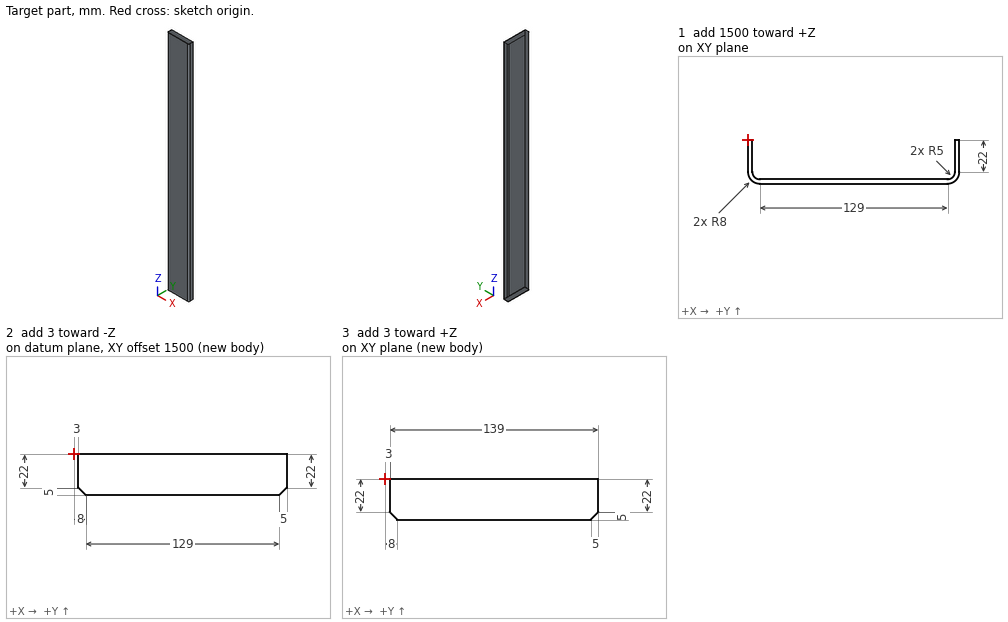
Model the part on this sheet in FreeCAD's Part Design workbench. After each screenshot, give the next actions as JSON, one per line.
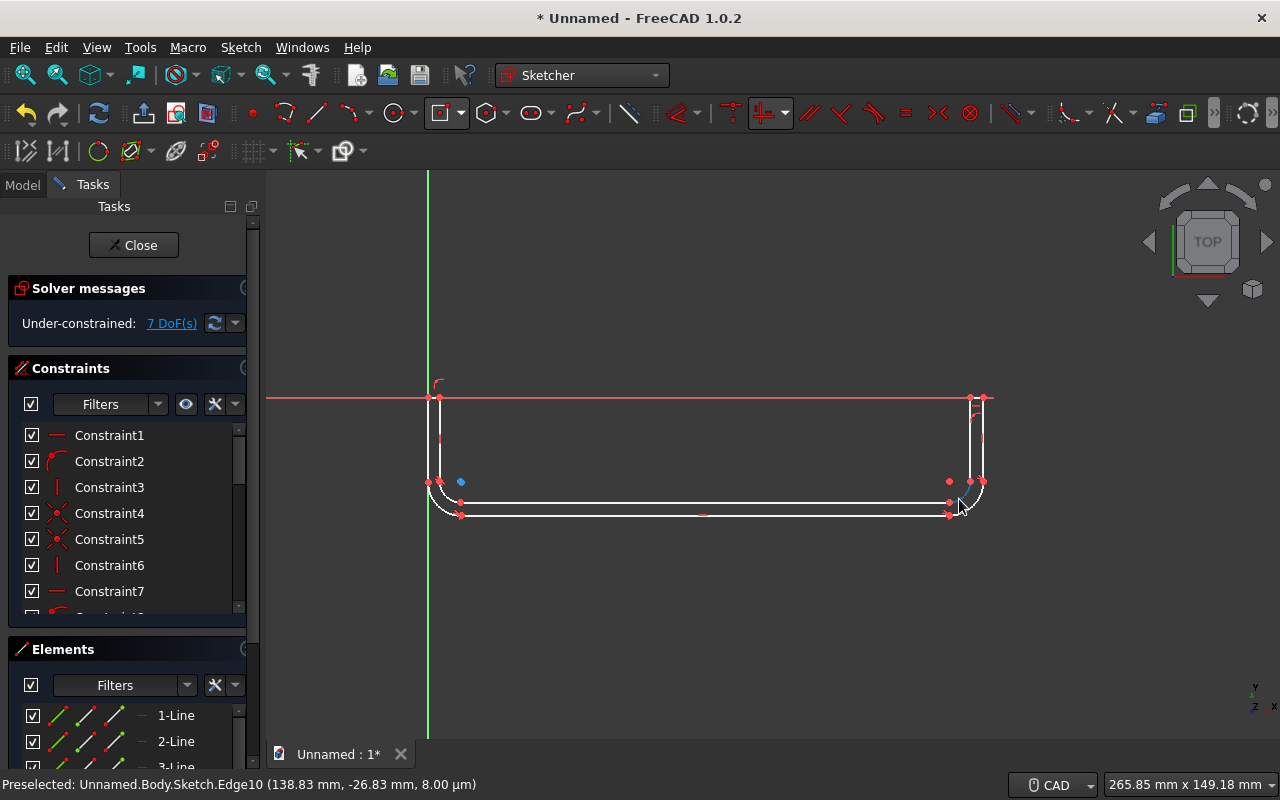
{"action": "scroll", "coordinate": [442, 491], "scroll_direction": "up", "scroll_amount": 2}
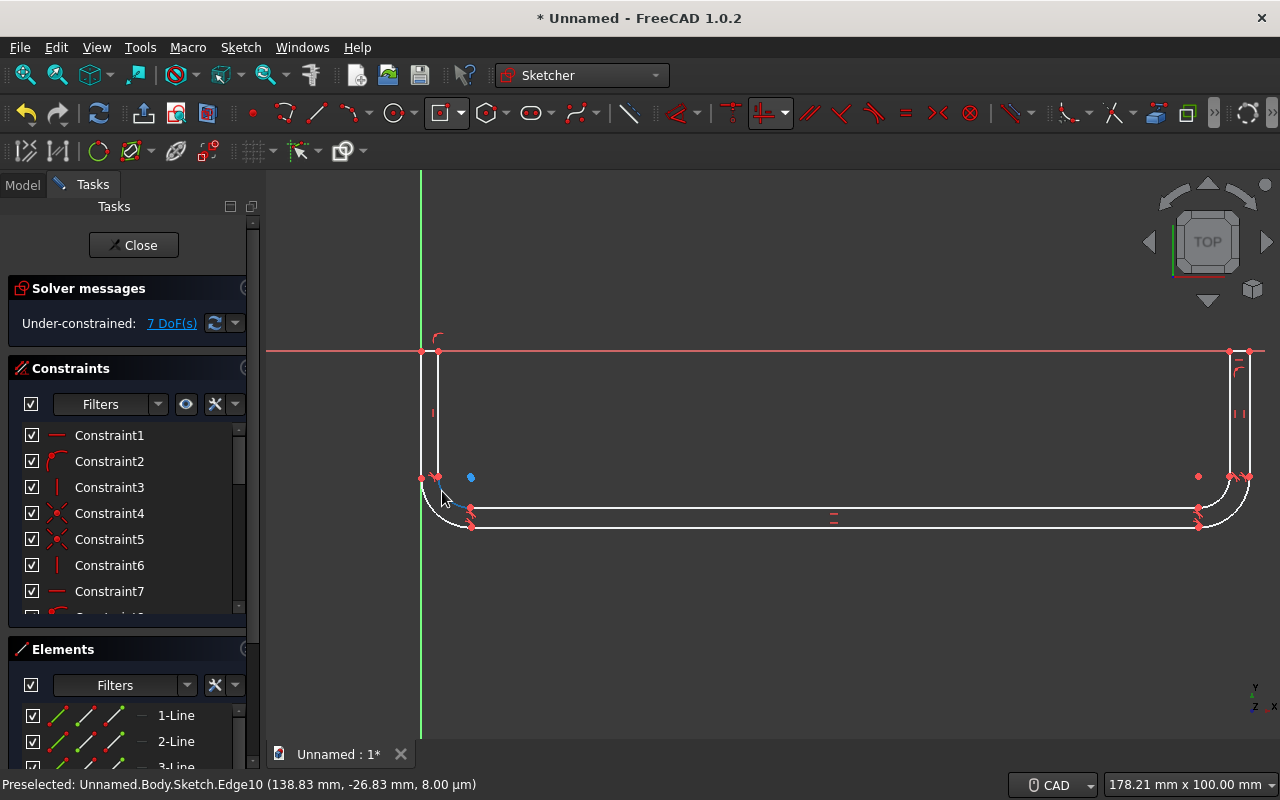
{"action": "left_click", "coordinate": [442, 490]}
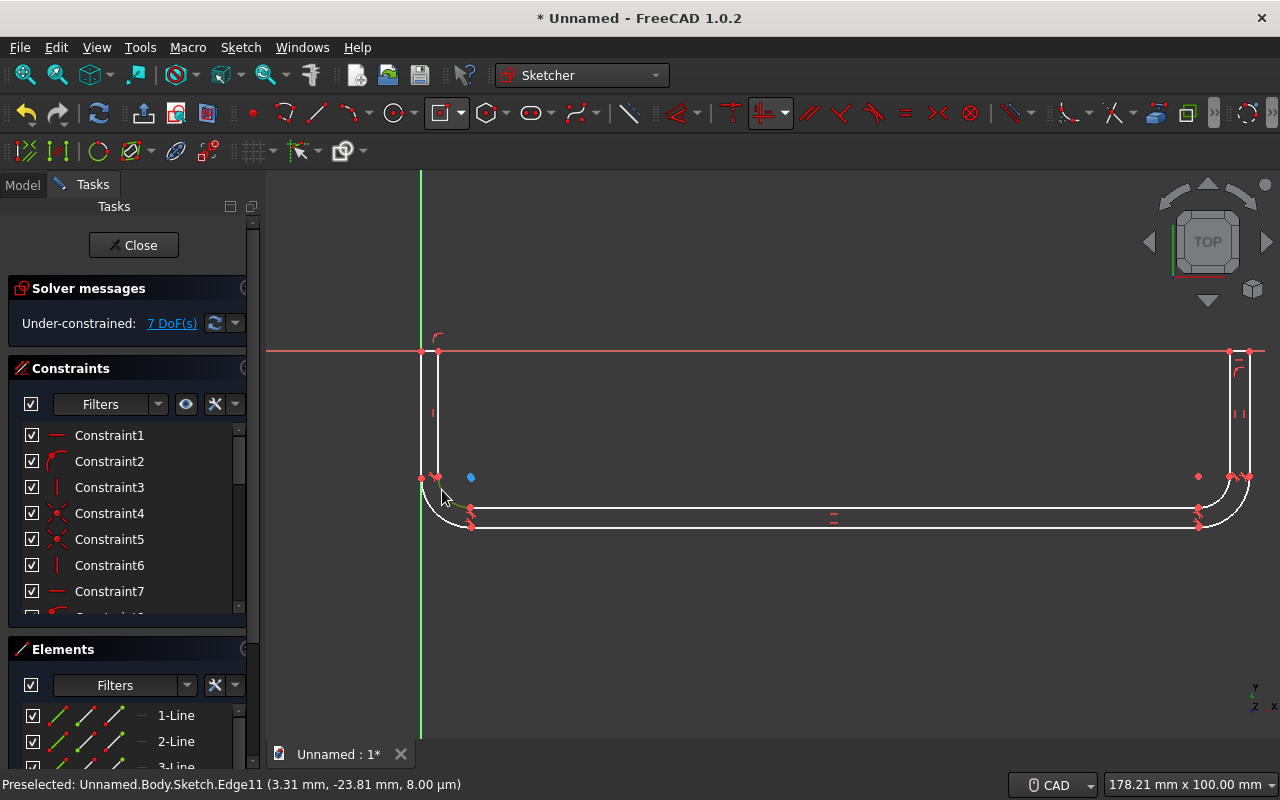
{"action": "left_click", "coordinate": [448, 522]}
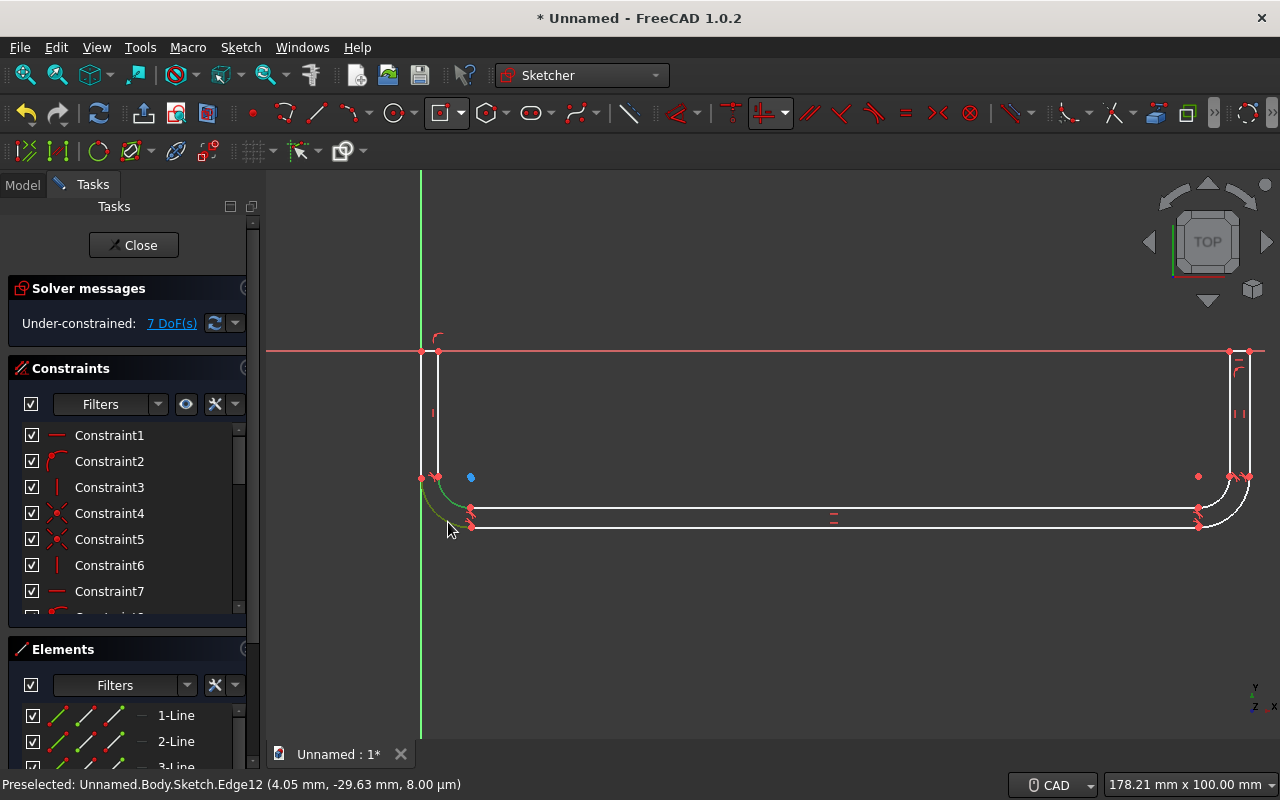
{"action": "left_click", "coordinate": [732, 114]}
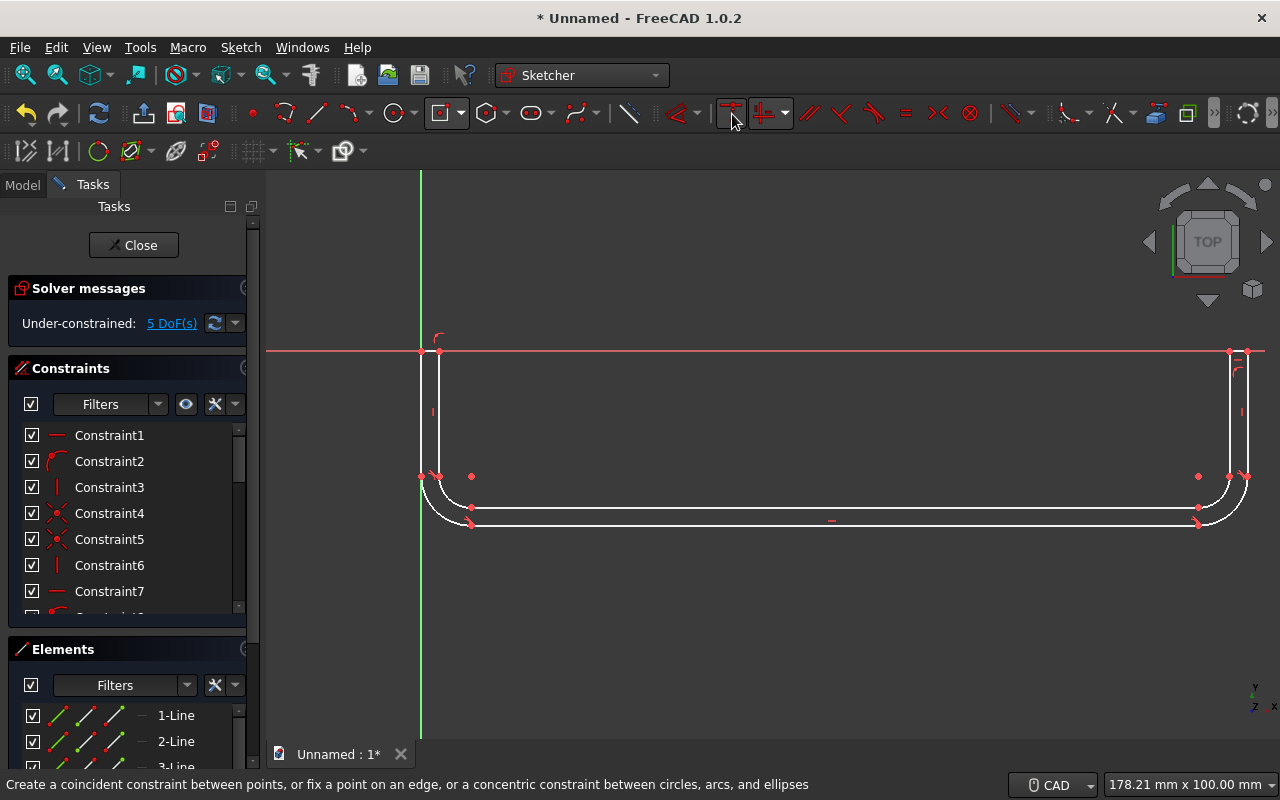
{"action": "scroll", "coordinate": [441, 491], "scroll_direction": "down", "scroll_amount": 2}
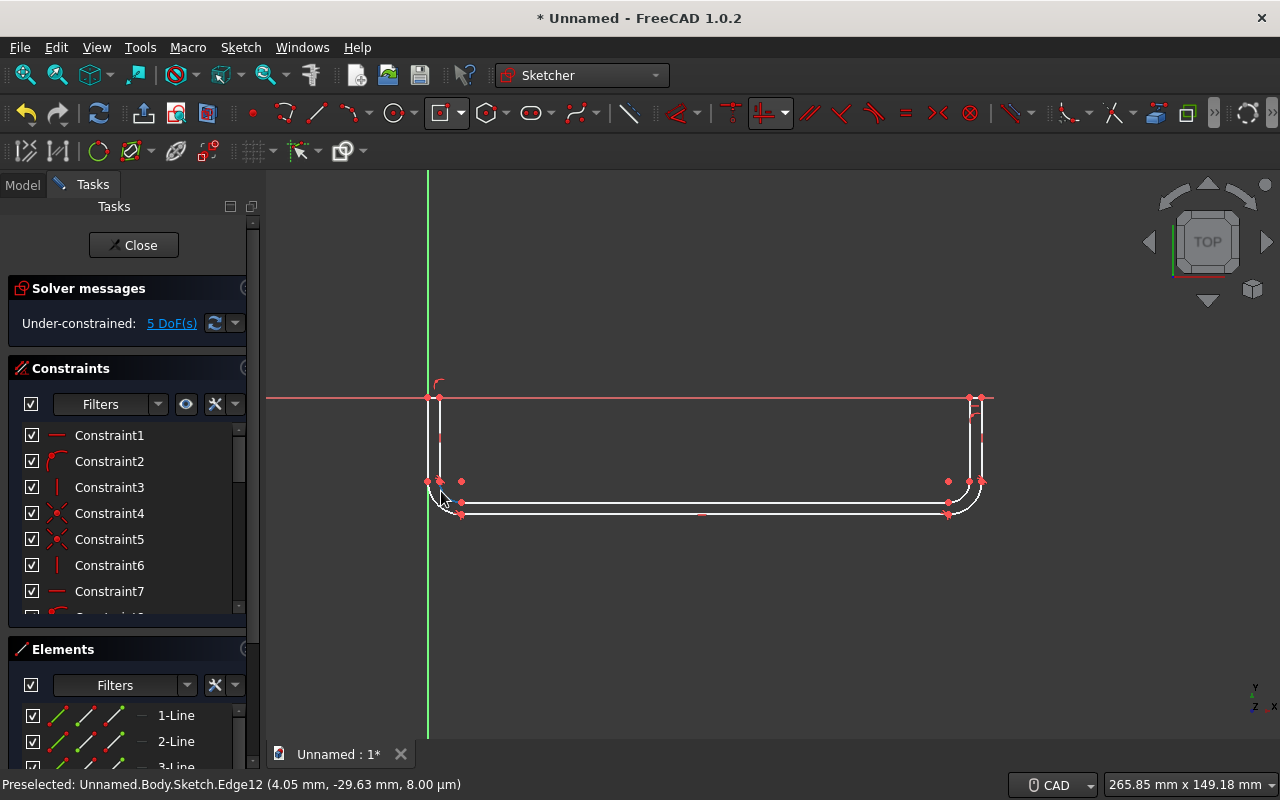
{"action": "scroll", "coordinate": [958, 500], "scroll_direction": "up", "scroll_amount": 2}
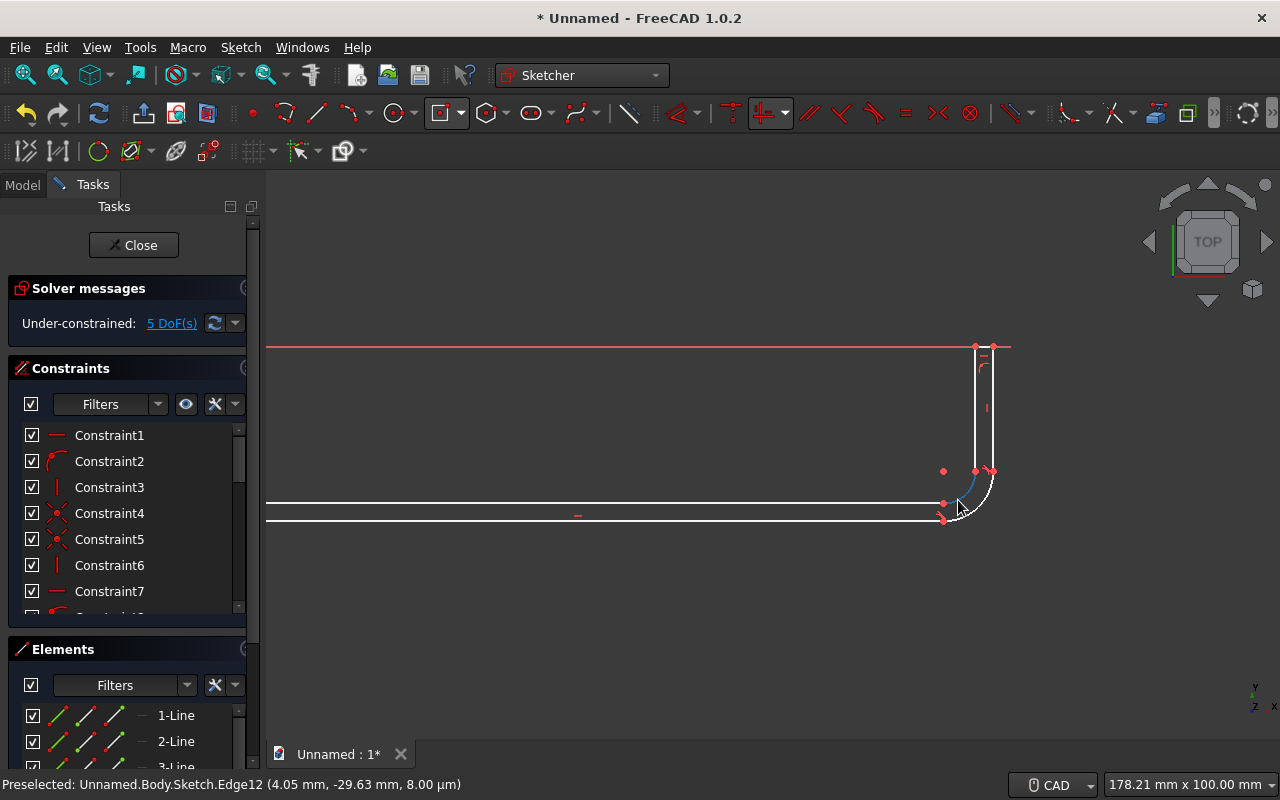
{"action": "left_click", "coordinate": [958, 500]}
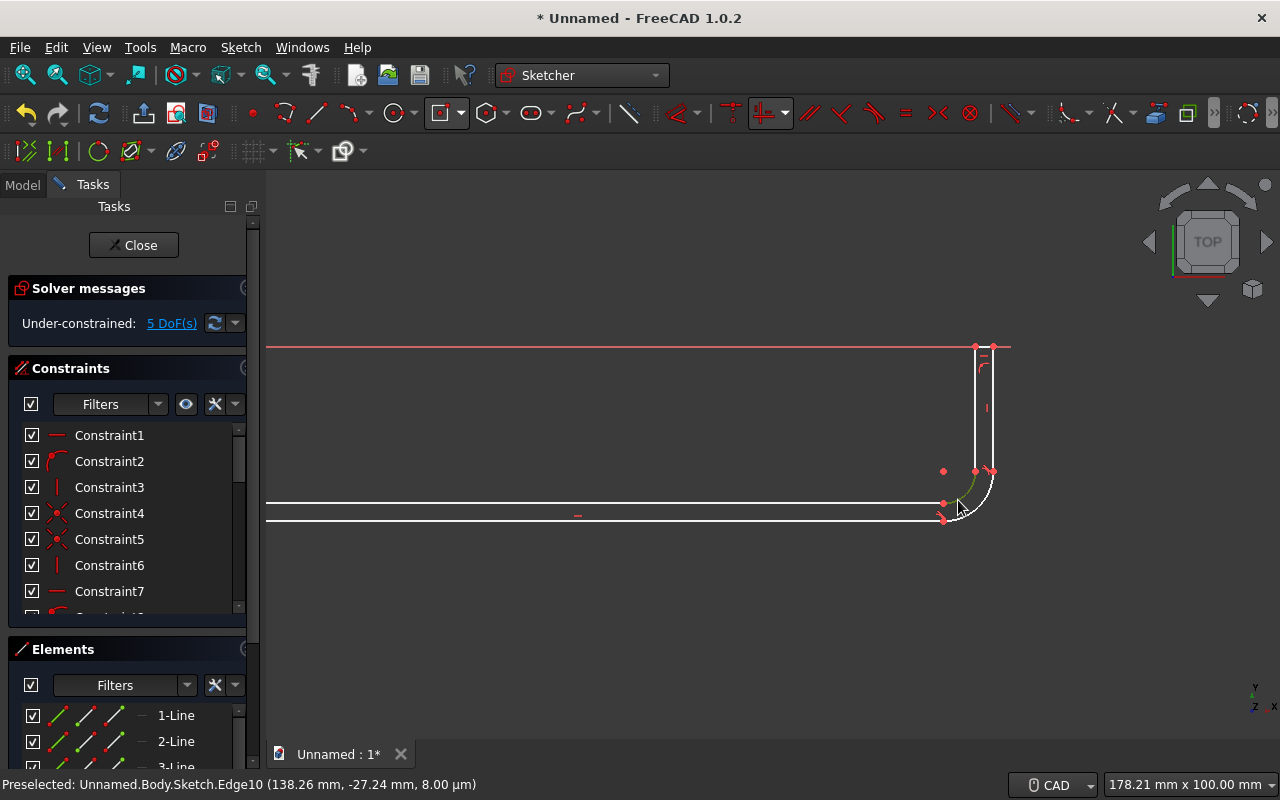
{"action": "scroll", "coordinate": [959, 500], "scroll_direction": "down", "scroll_amount": 2}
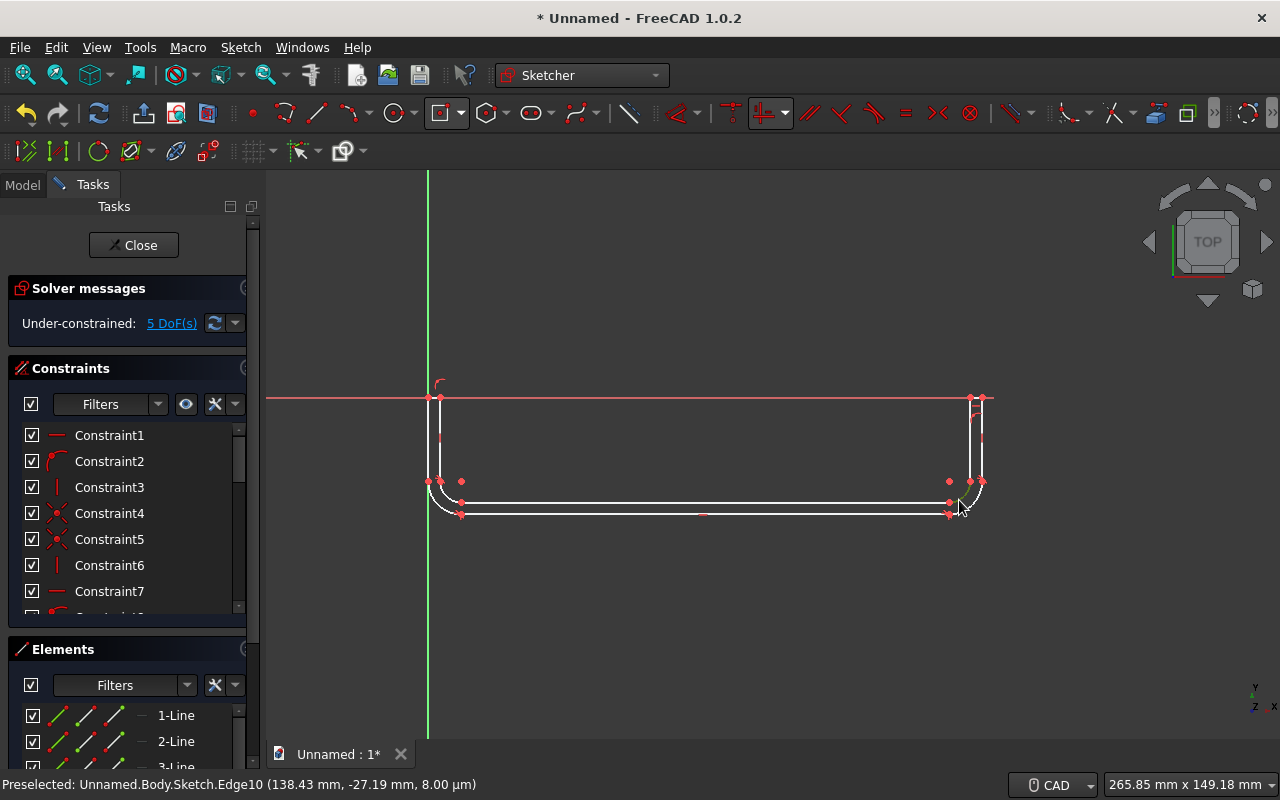
{"action": "scroll", "coordinate": [442, 491], "scroll_direction": "up", "scroll_amount": 2}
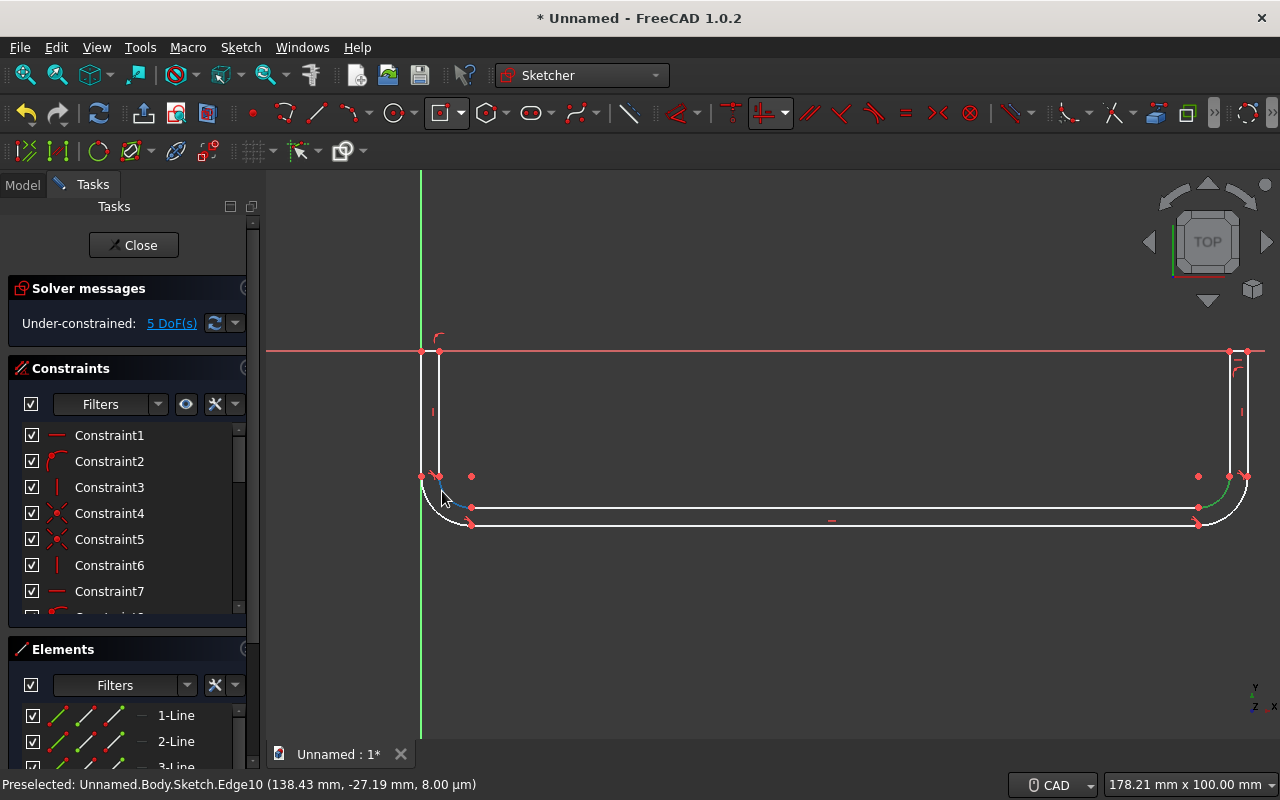
{"action": "left_click", "coordinate": [443, 490]}